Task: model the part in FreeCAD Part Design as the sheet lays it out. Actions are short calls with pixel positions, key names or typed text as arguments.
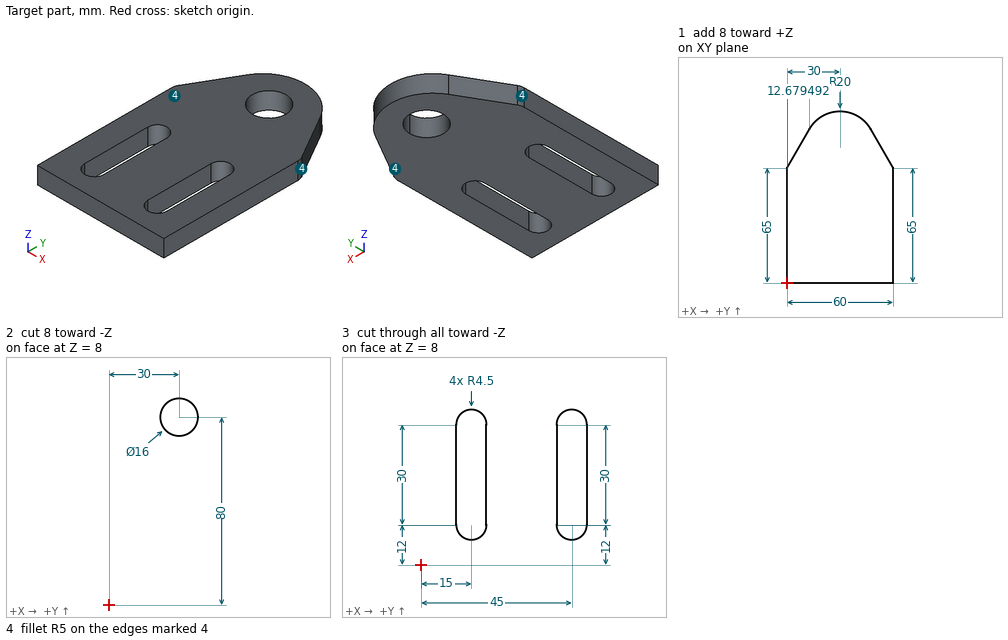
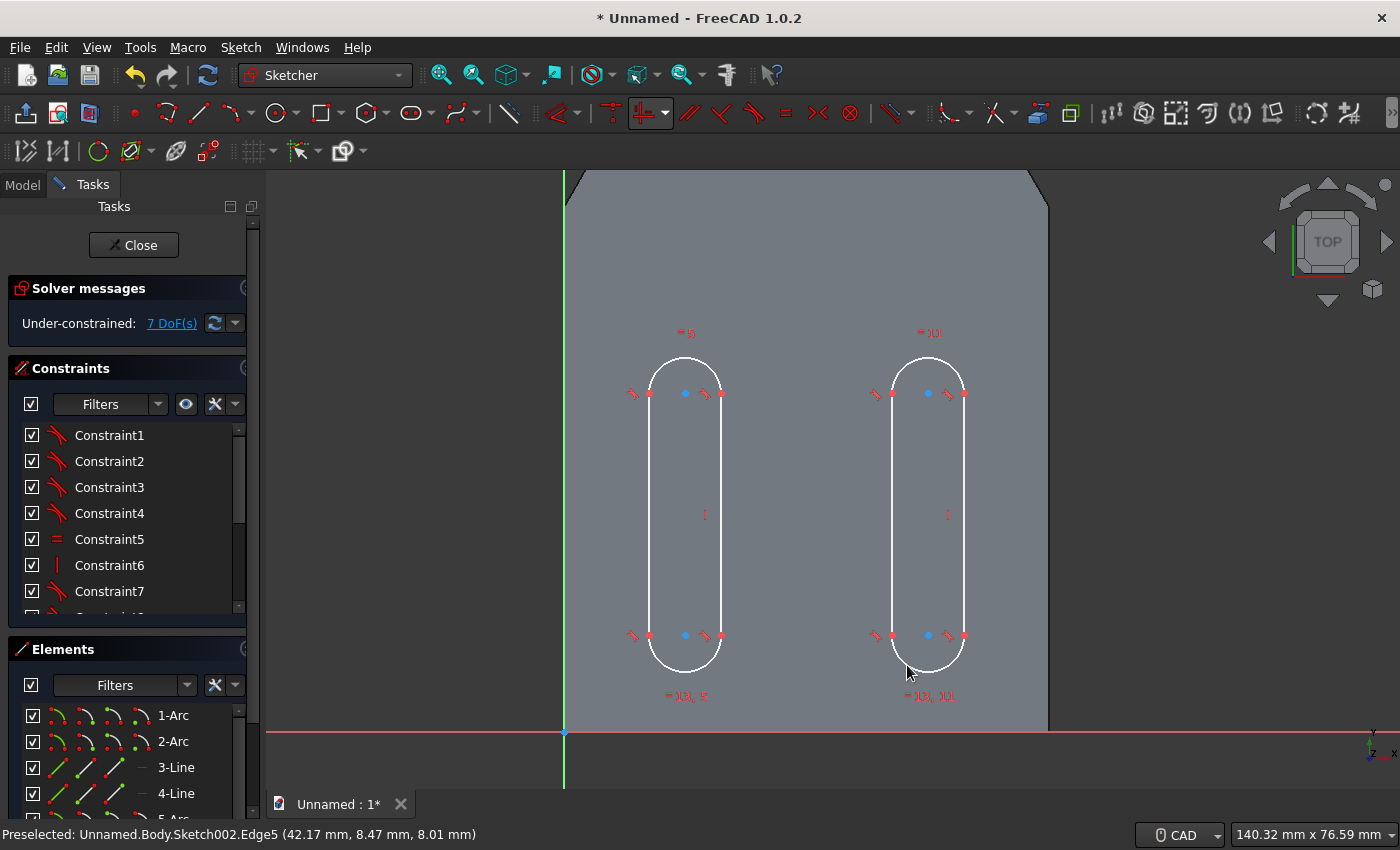
key(d)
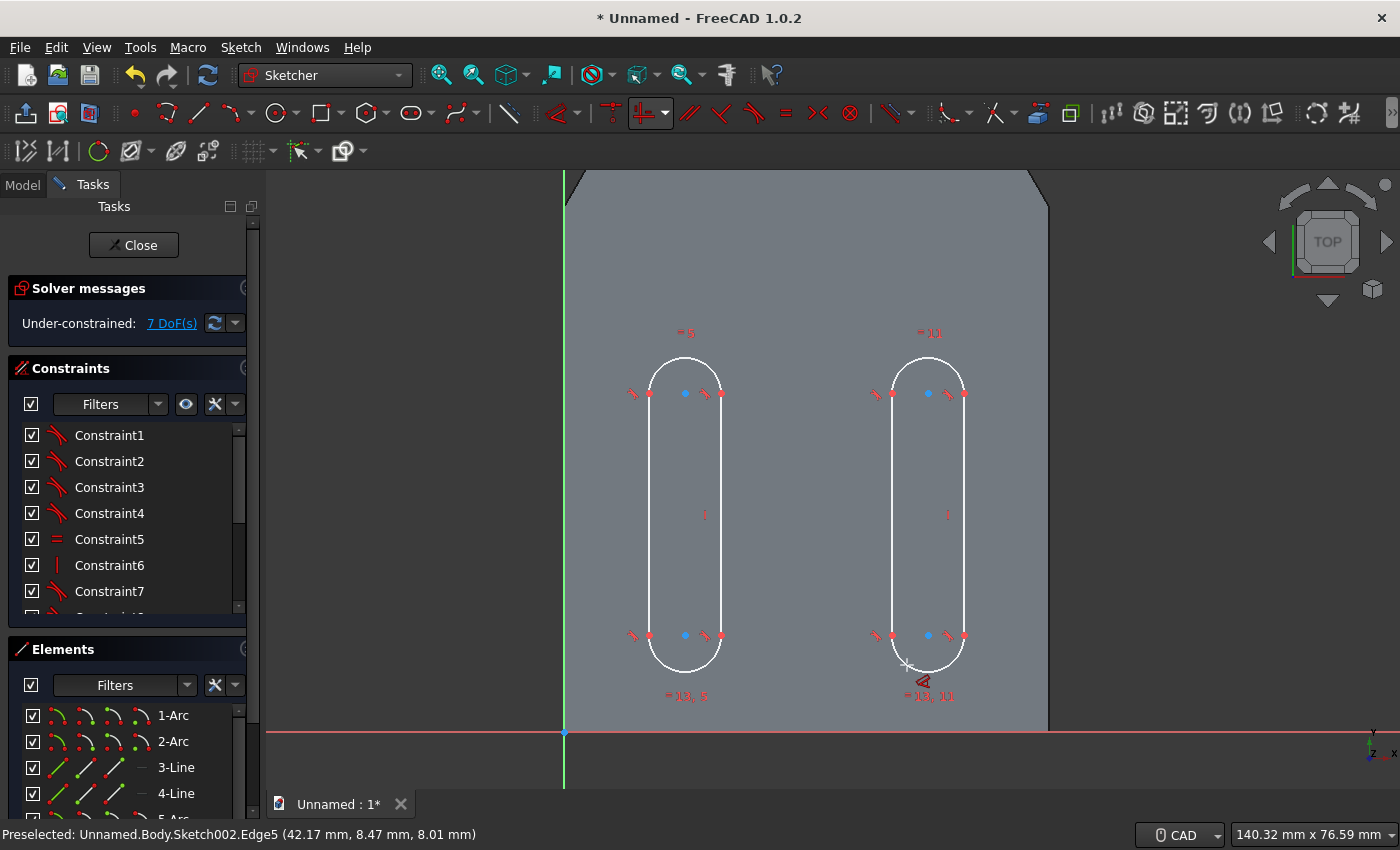
click(664, 665)
click(645, 691)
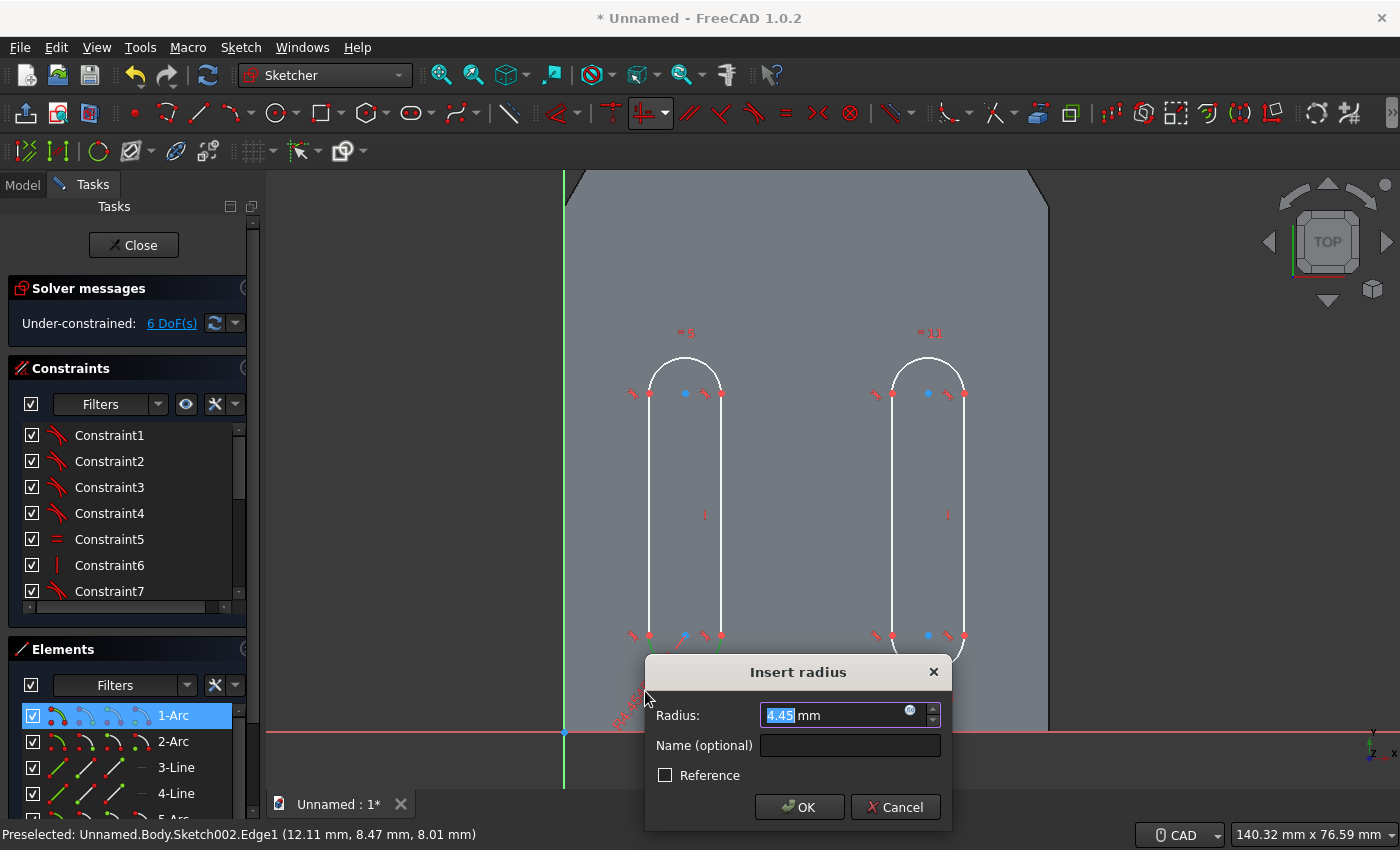
text(4.5)
key(Return)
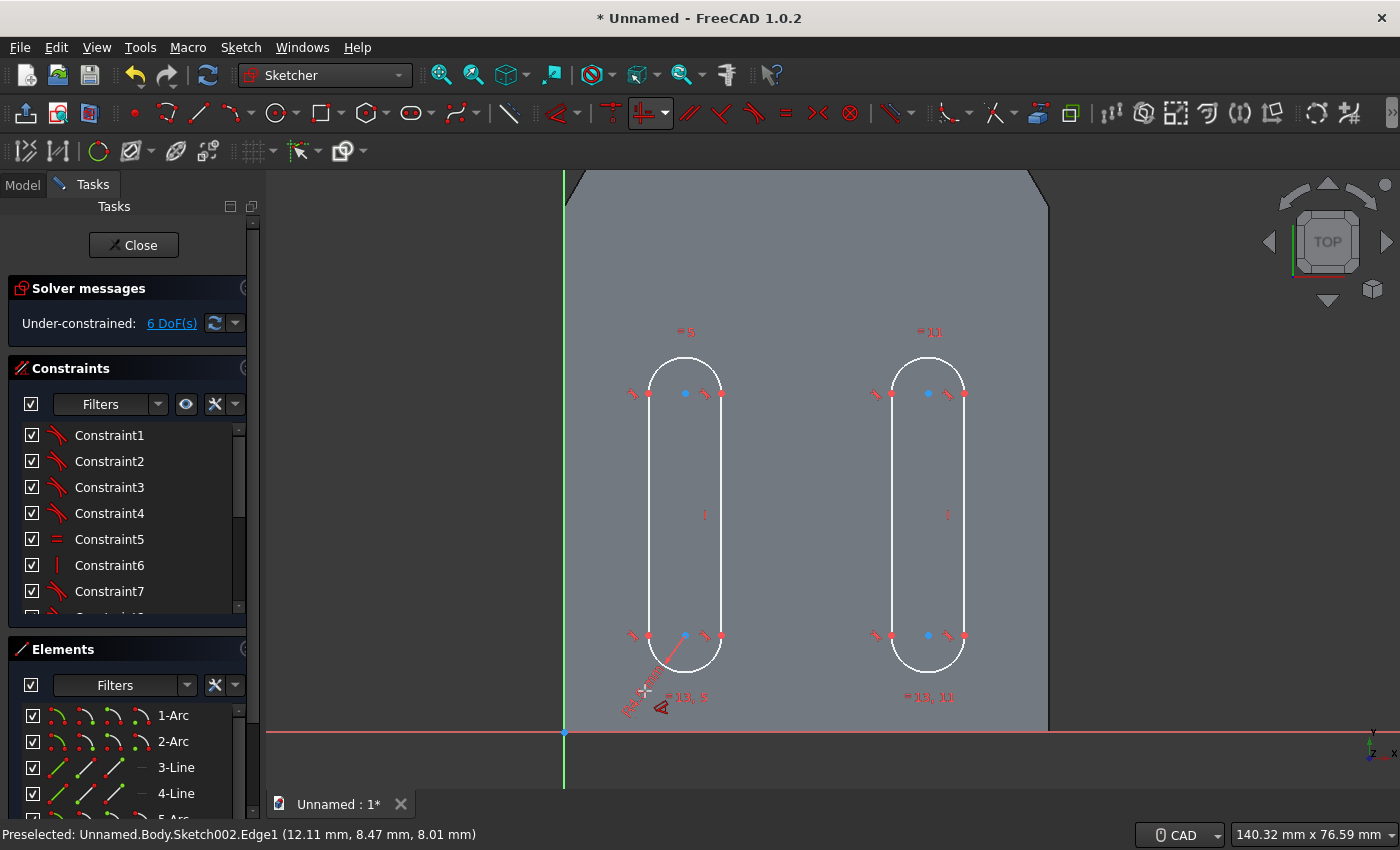
click(649, 563)
click(615, 515)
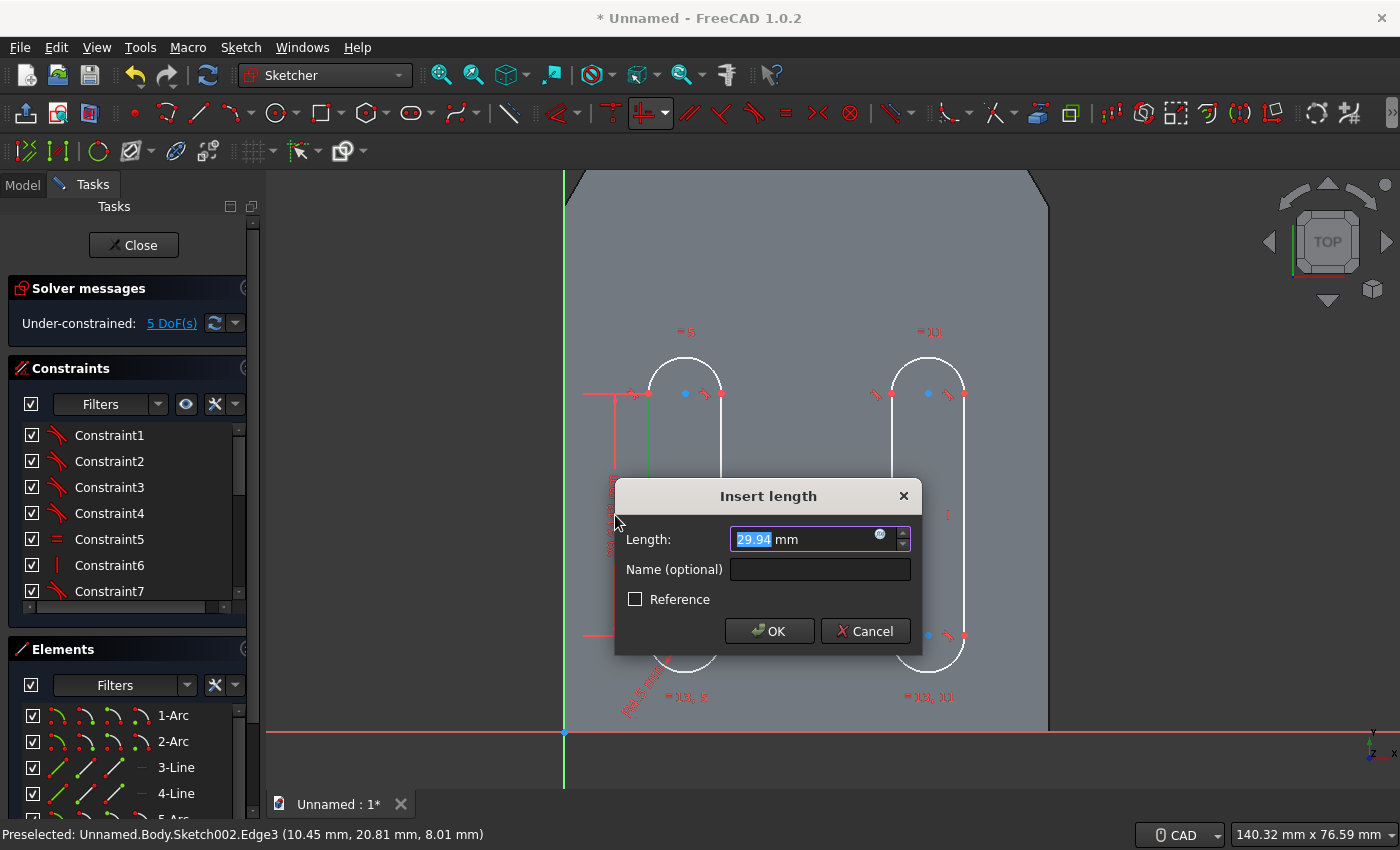
text(30)
key(Return)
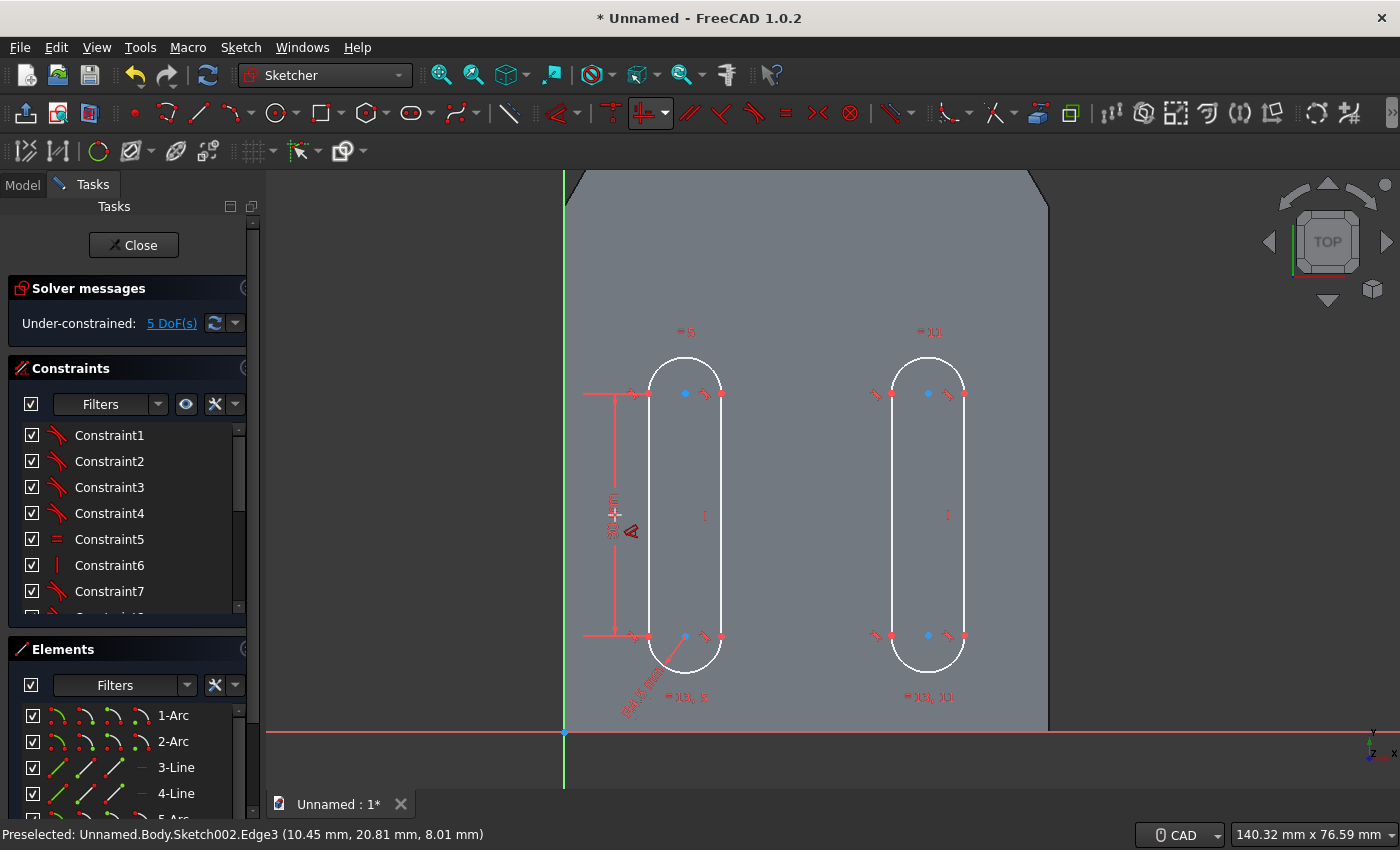
click(892, 563)
click(926, 515)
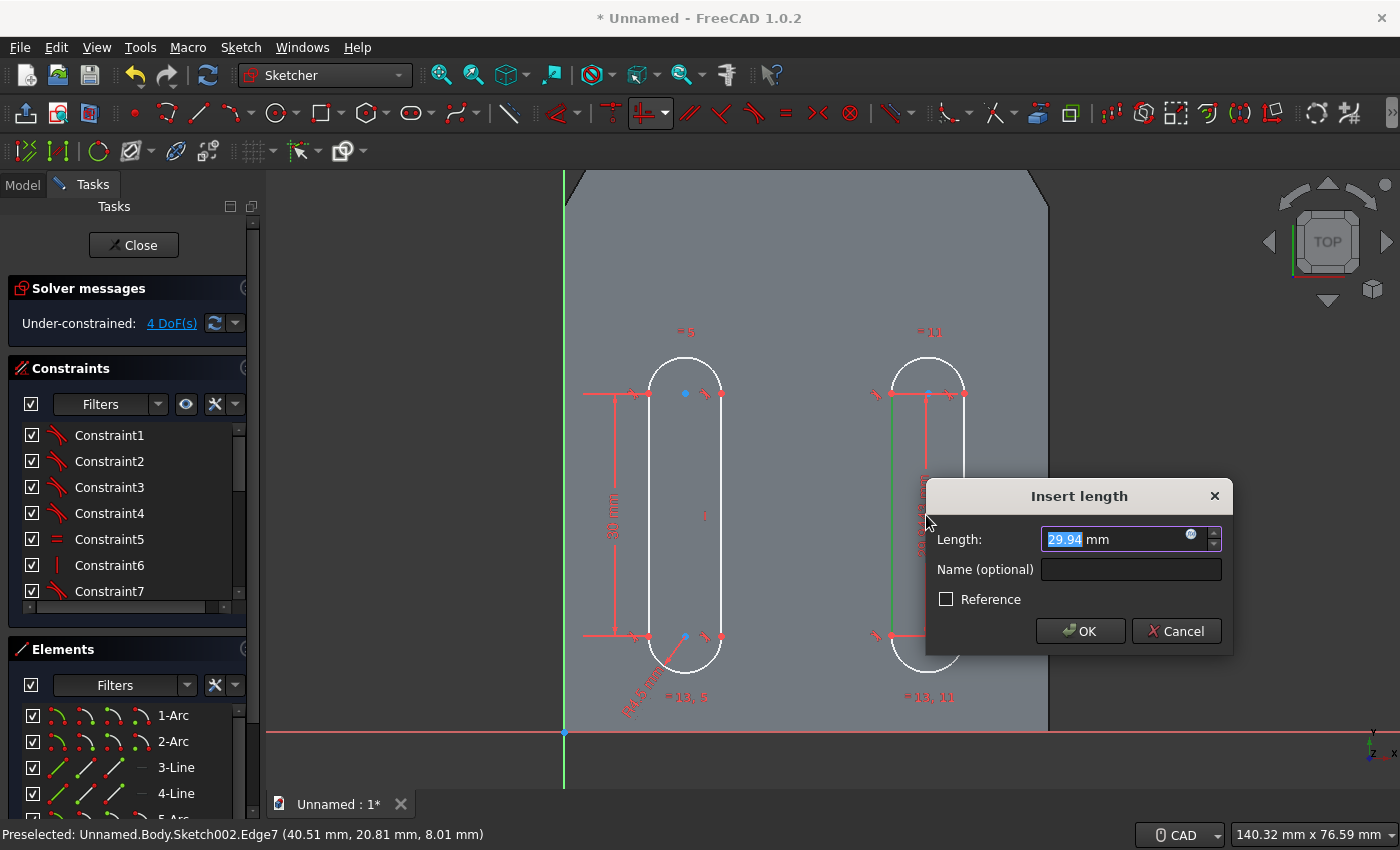
text(30)
key(Return)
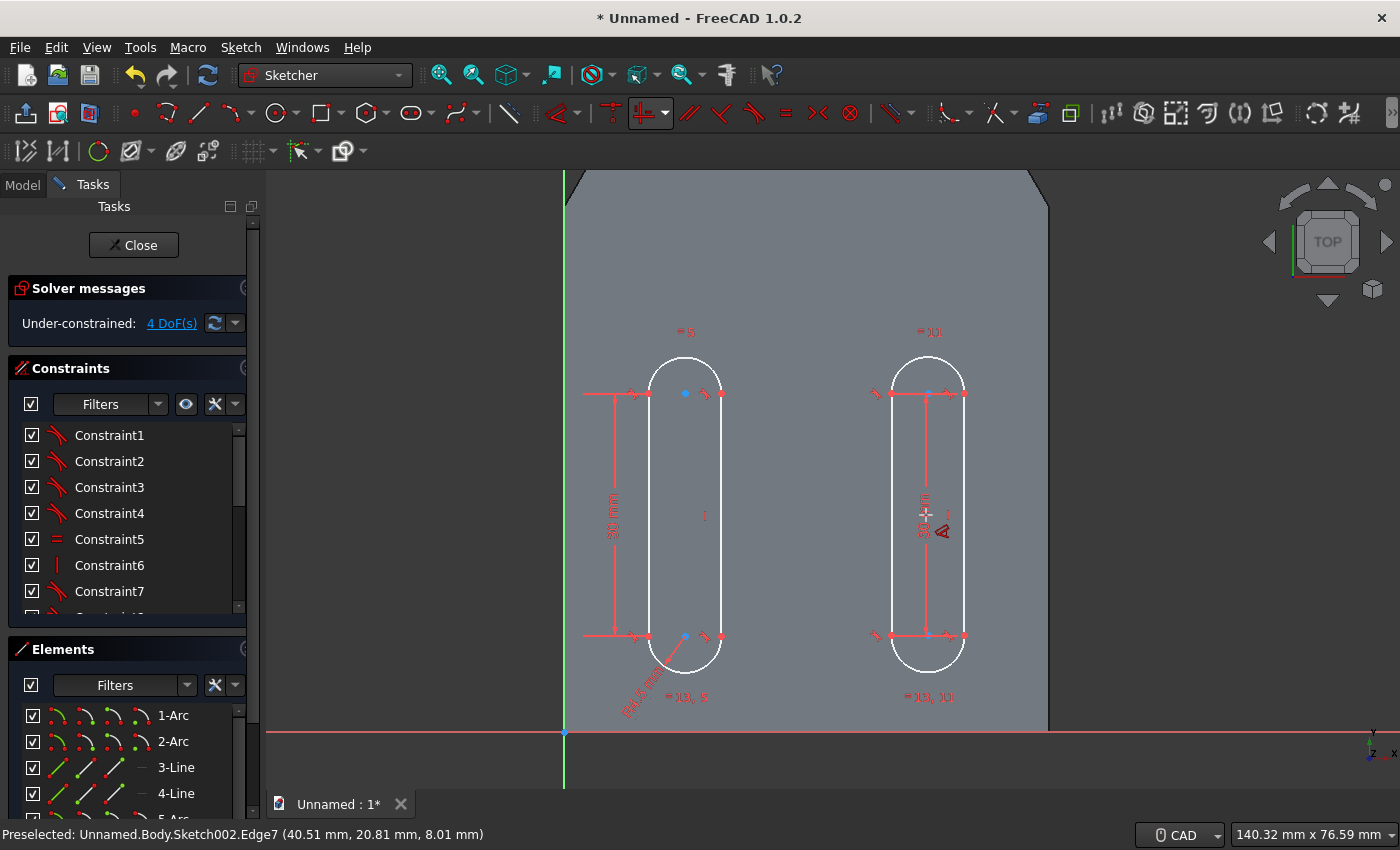
click(649, 636)
click(530, 684)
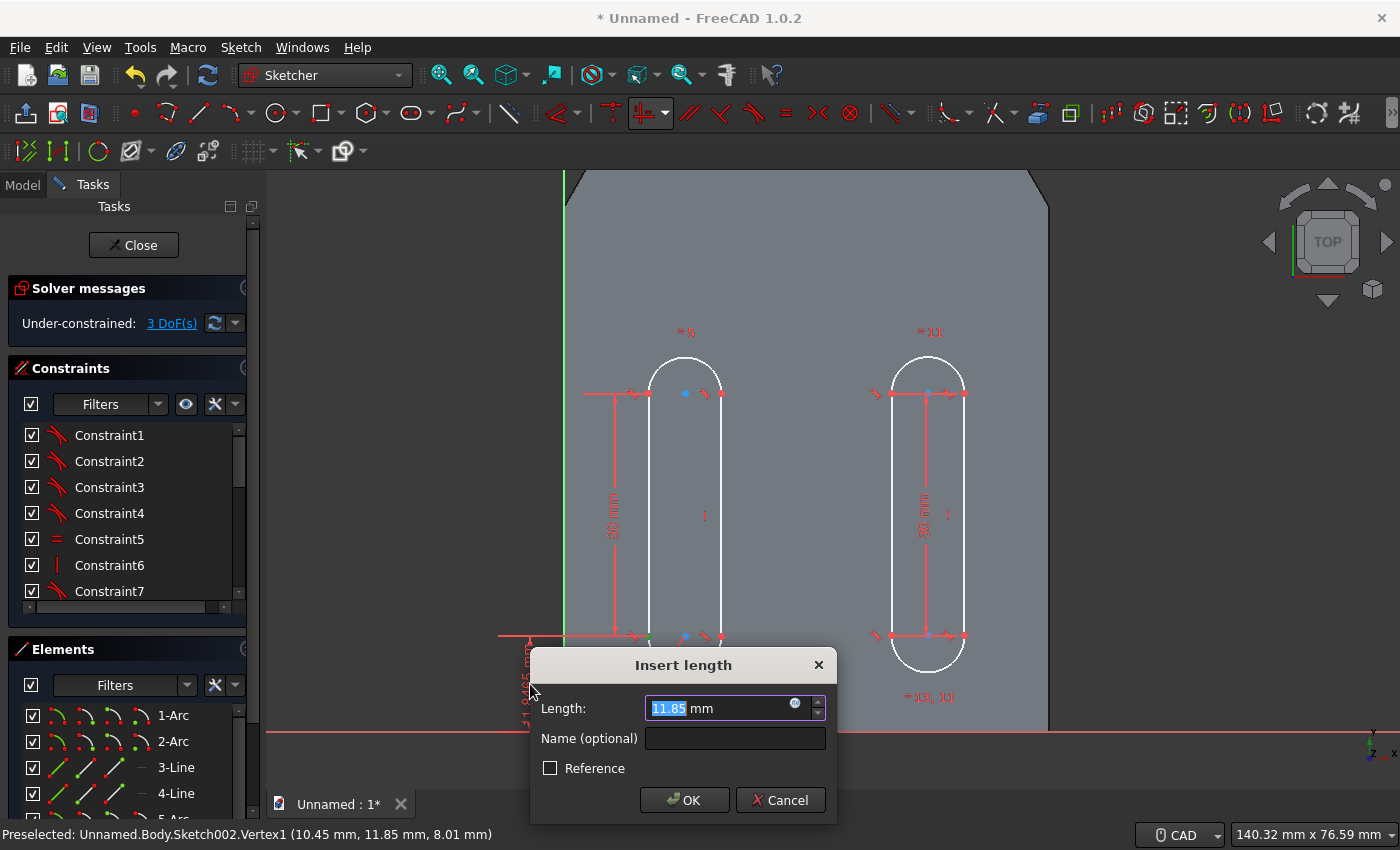
text(12)
key(Return)